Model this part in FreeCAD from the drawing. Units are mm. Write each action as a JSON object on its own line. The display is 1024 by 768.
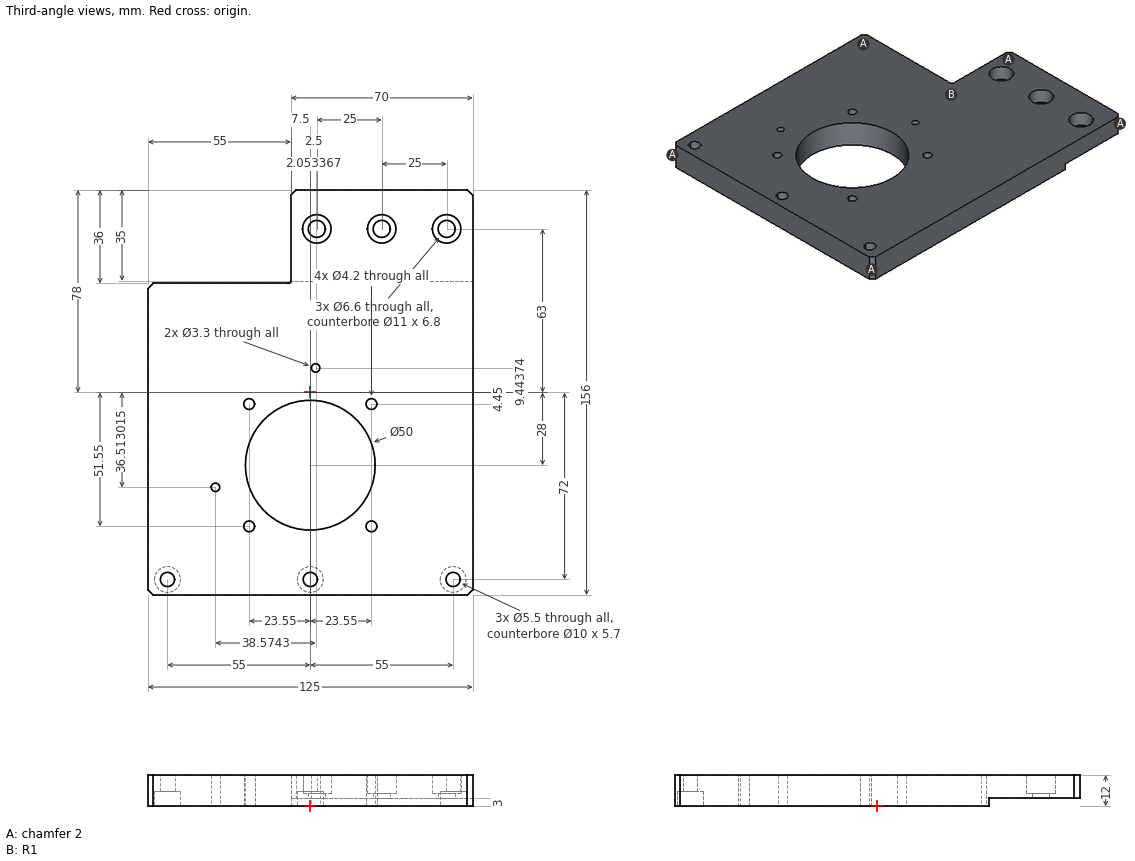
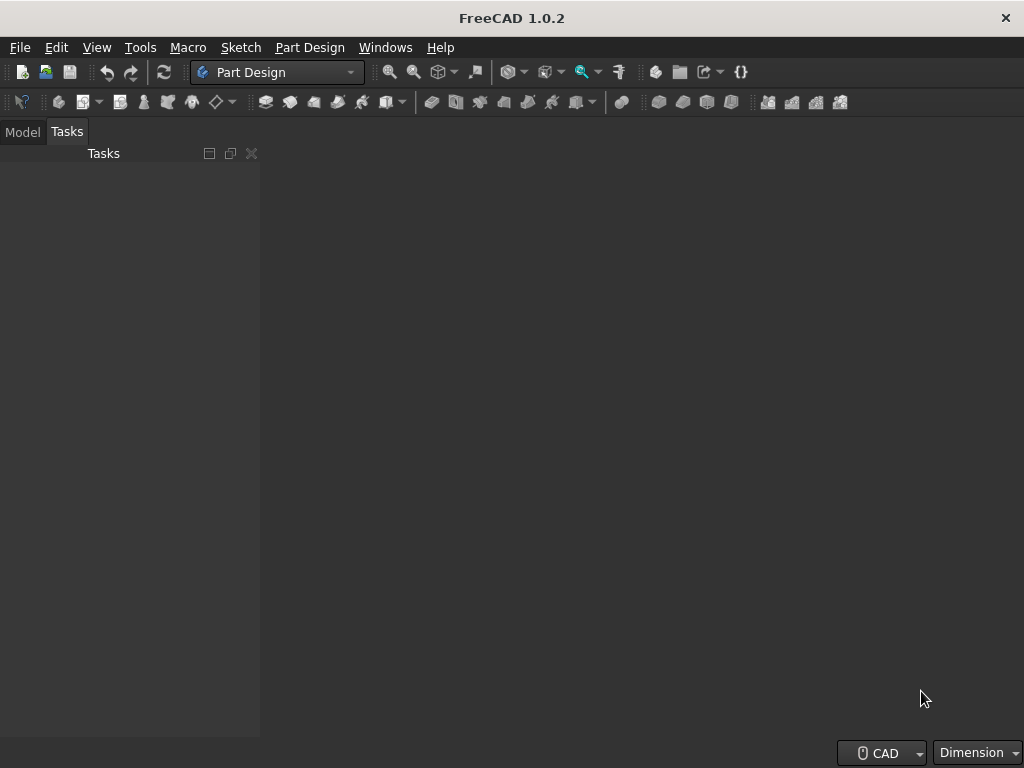
{"action": "left_click", "coordinate": [22, 72]}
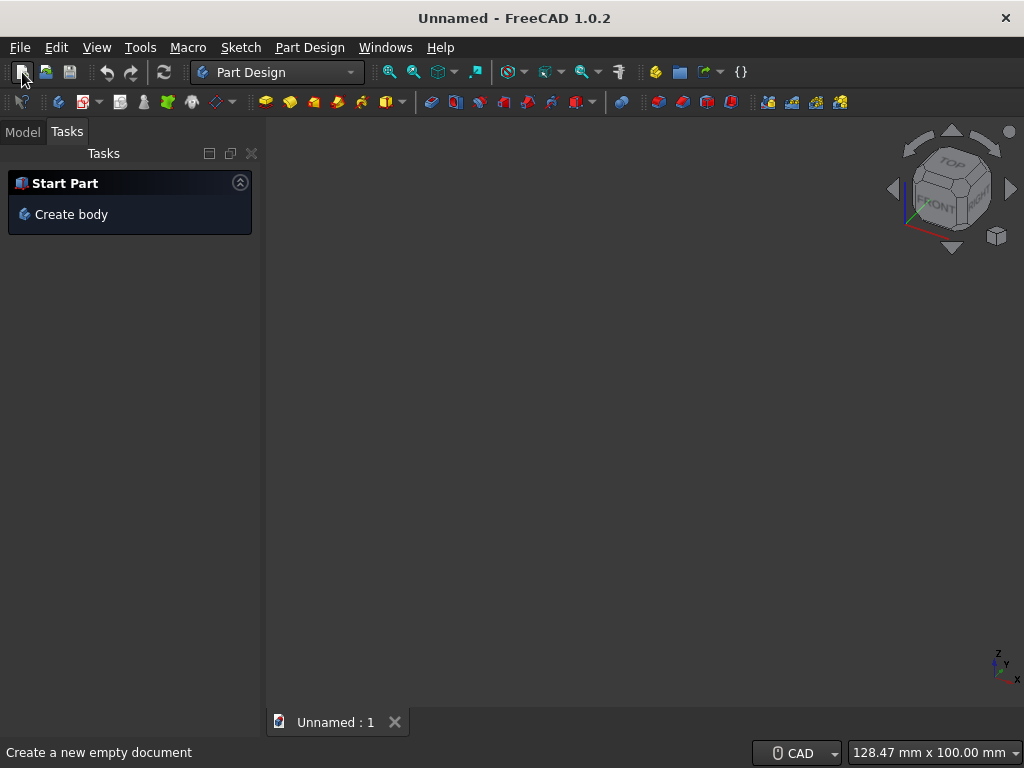
{"action": "left_click", "coordinate": [84, 102]}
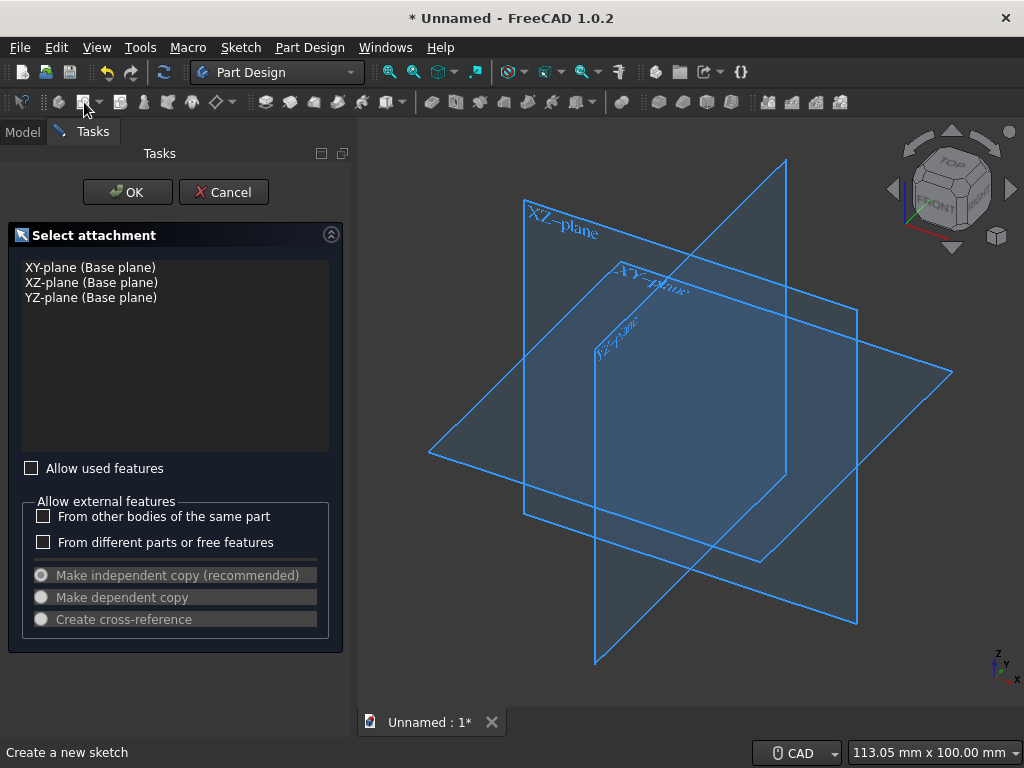
{"action": "left_click", "coordinate": [82, 268]}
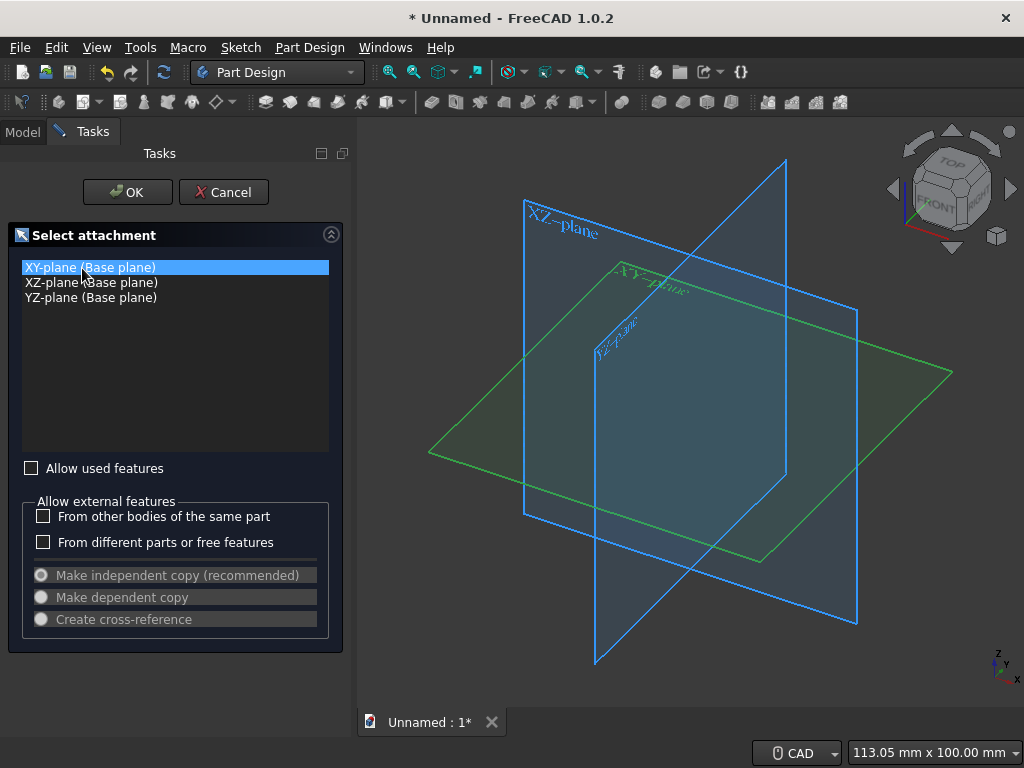
{"action": "left_click", "coordinate": [128, 192]}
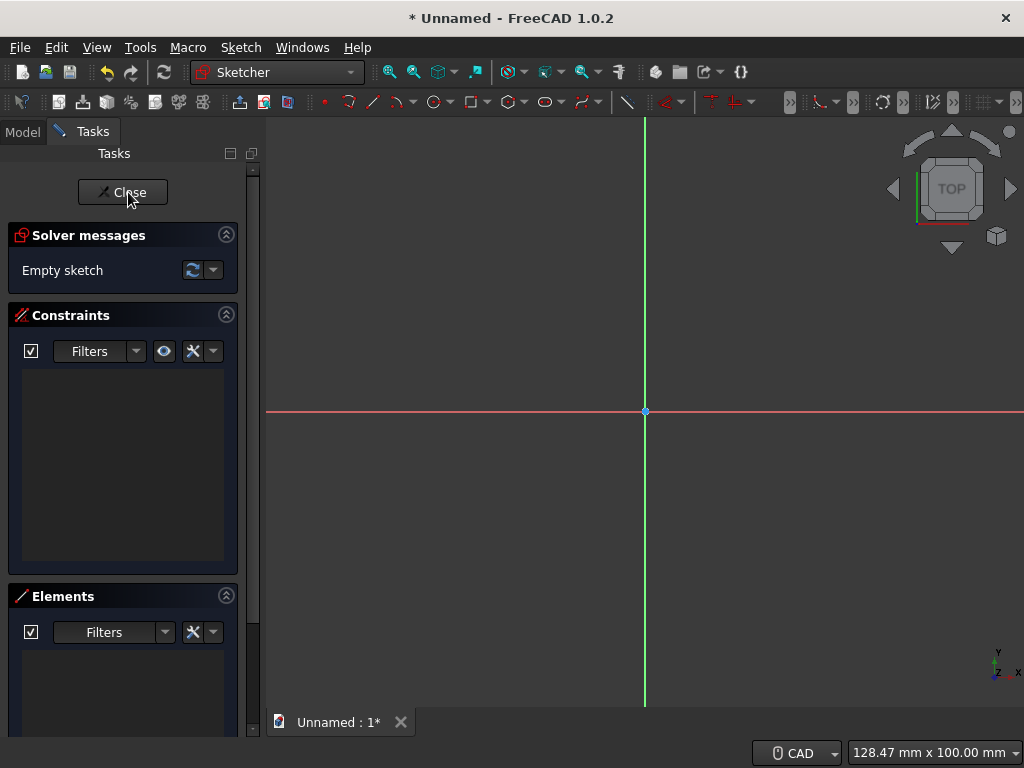
{"action": "scroll", "coordinate": [521, 412], "scroll_direction": "down", "scroll_amount": 4}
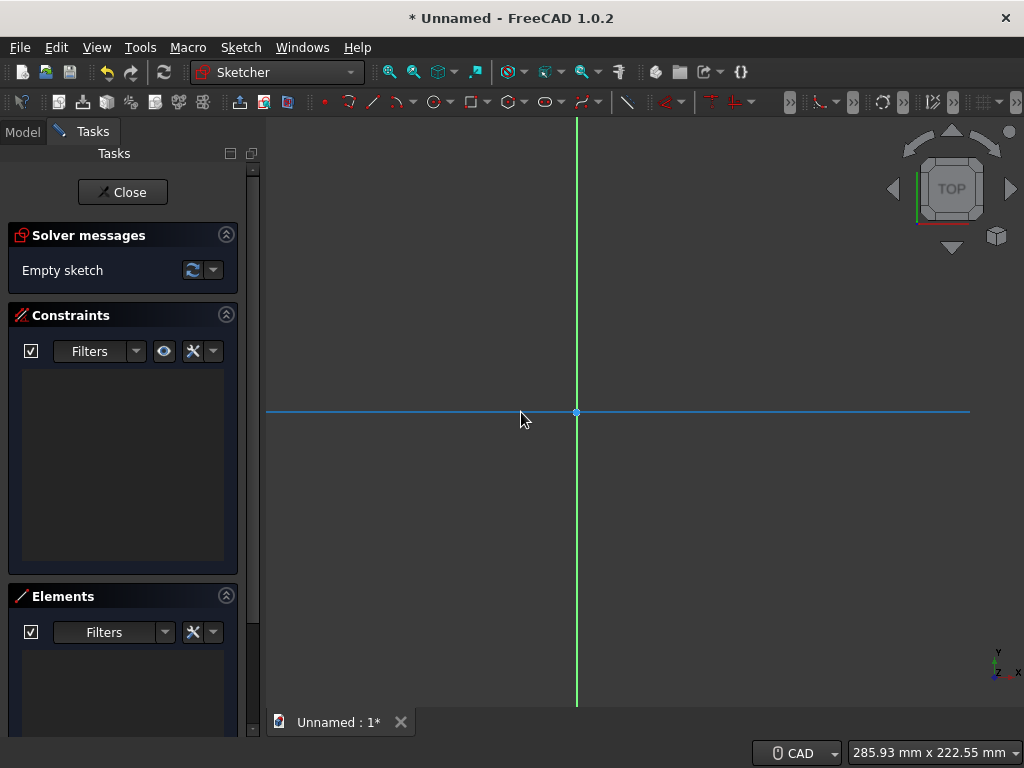
{"action": "left_click", "coordinate": [490, 102]}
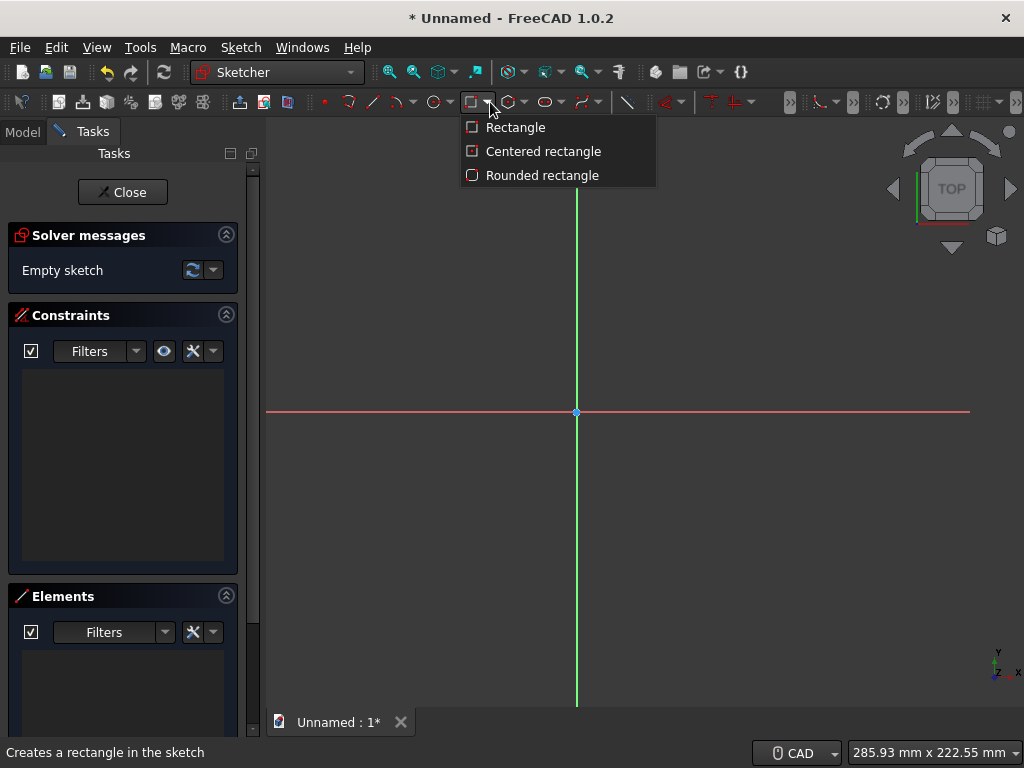
{"action": "left_click", "coordinate": [558, 151]}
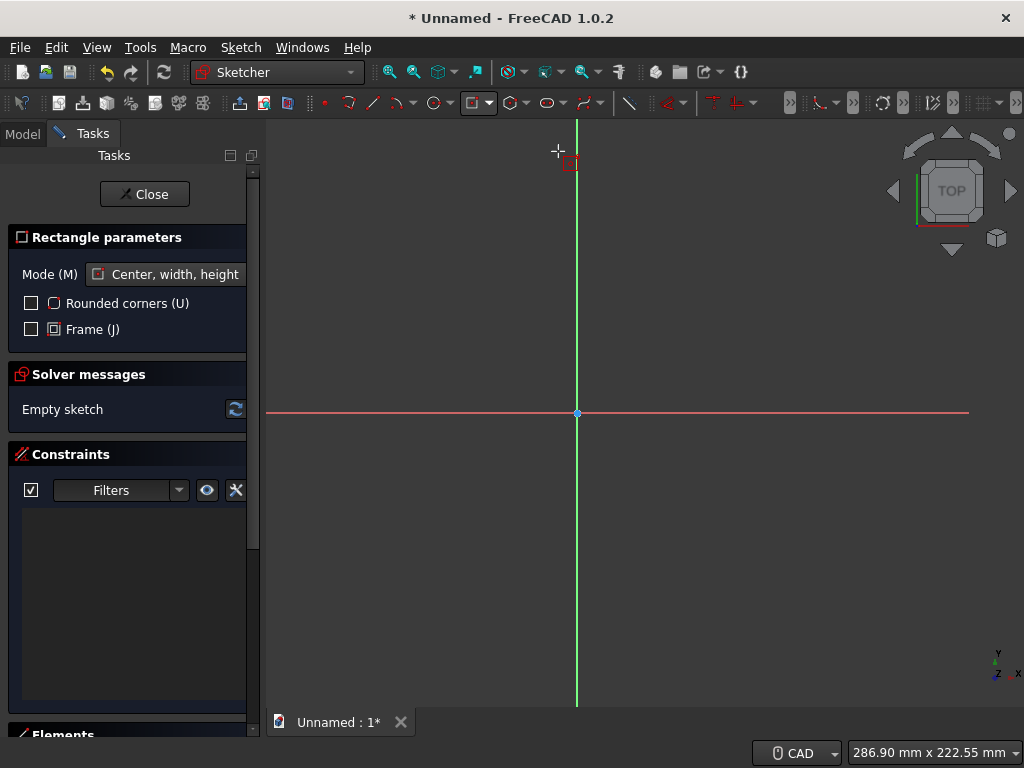
{"action": "left_click", "coordinate": [577, 413]}
{"action": "left_click", "coordinate": [742, 207]}
{"action": "key", "text": "Escape"}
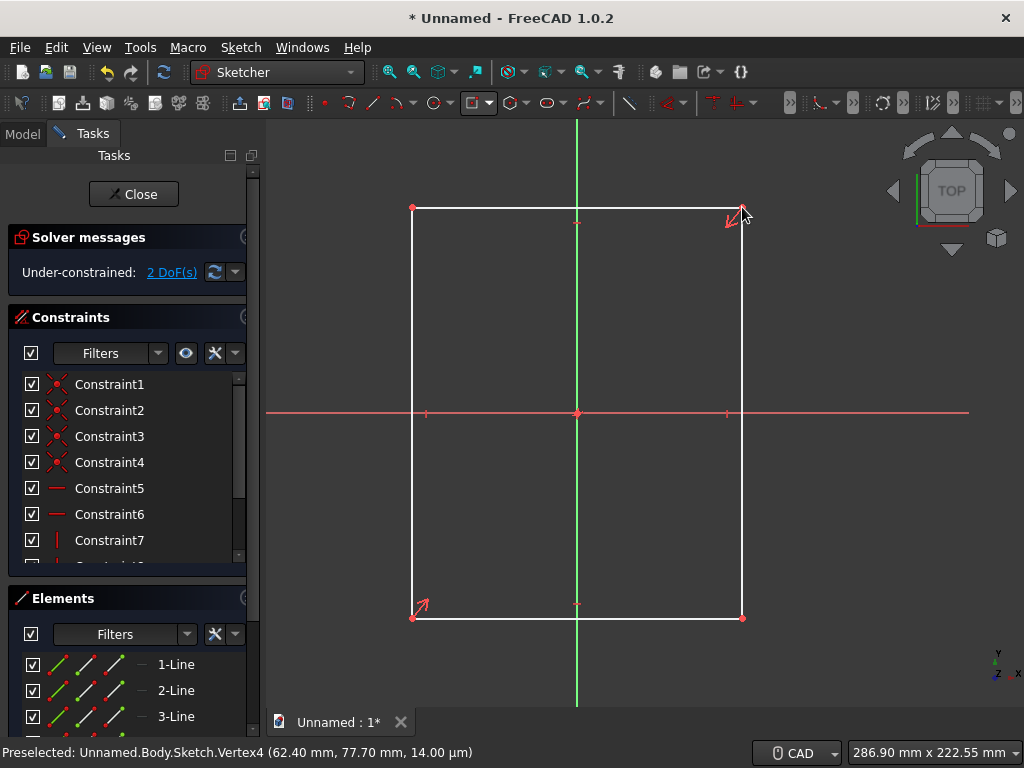
{"action": "left_click", "coordinate": [511, 619]}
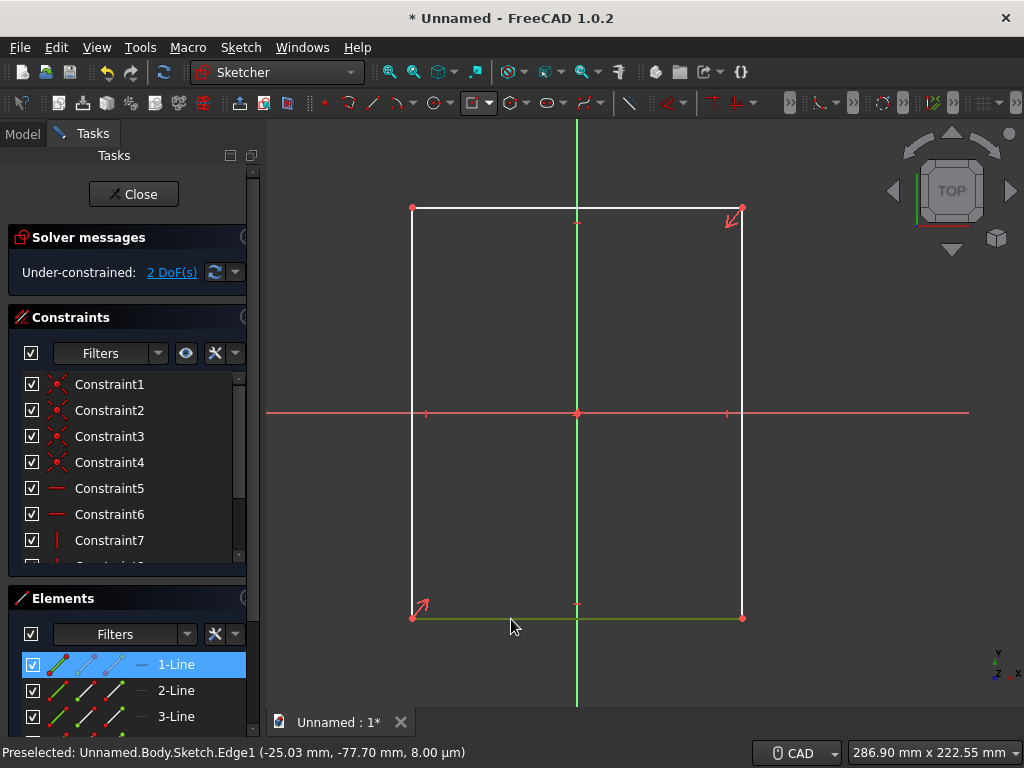
{"action": "left_click", "coordinate": [686, 104]}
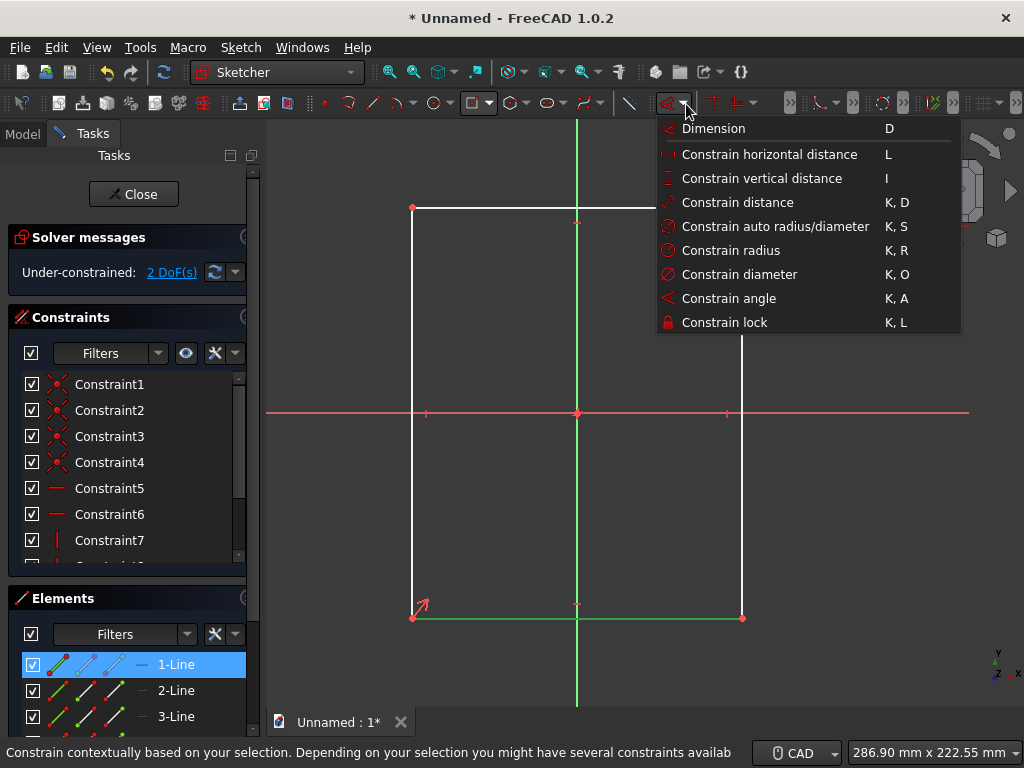
{"action": "left_click", "coordinate": [809, 154]}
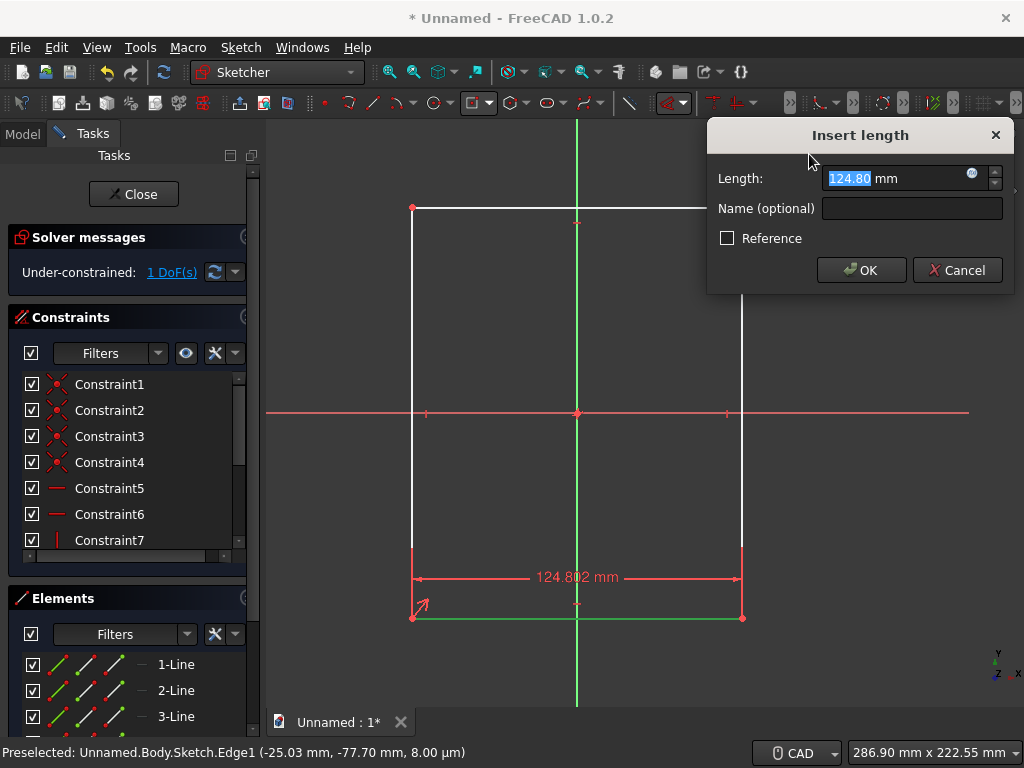
{"action": "type", "text": "125"}
{"action": "key", "text": "Return"}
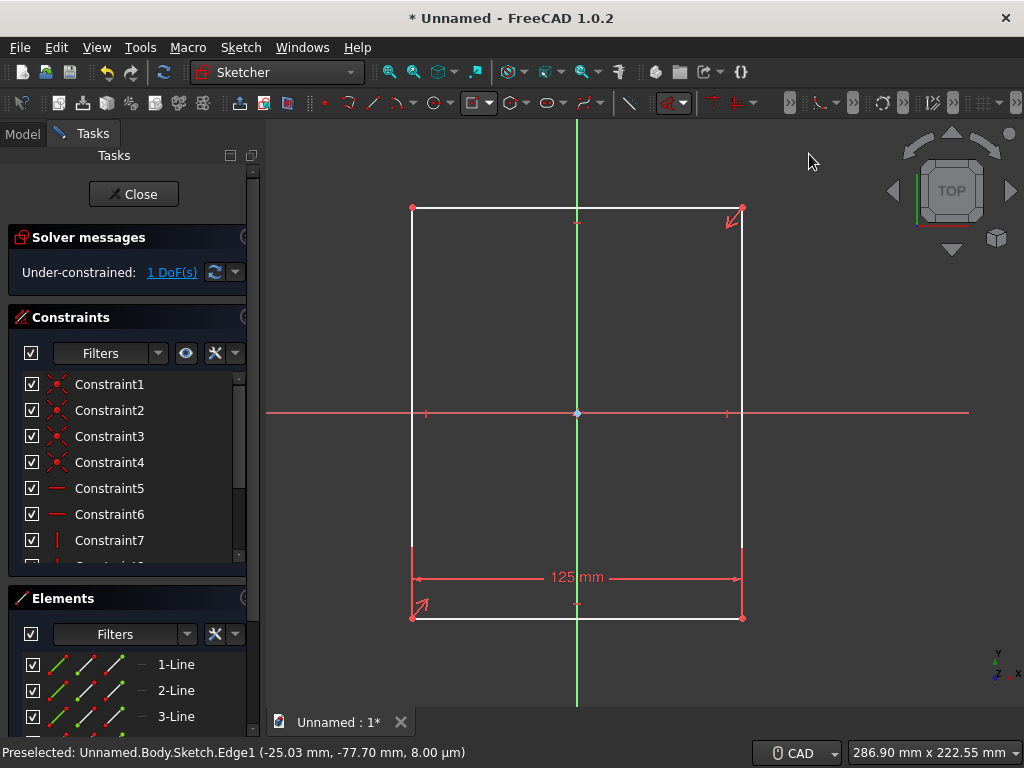
{"action": "left_click", "coordinate": [742, 495]}